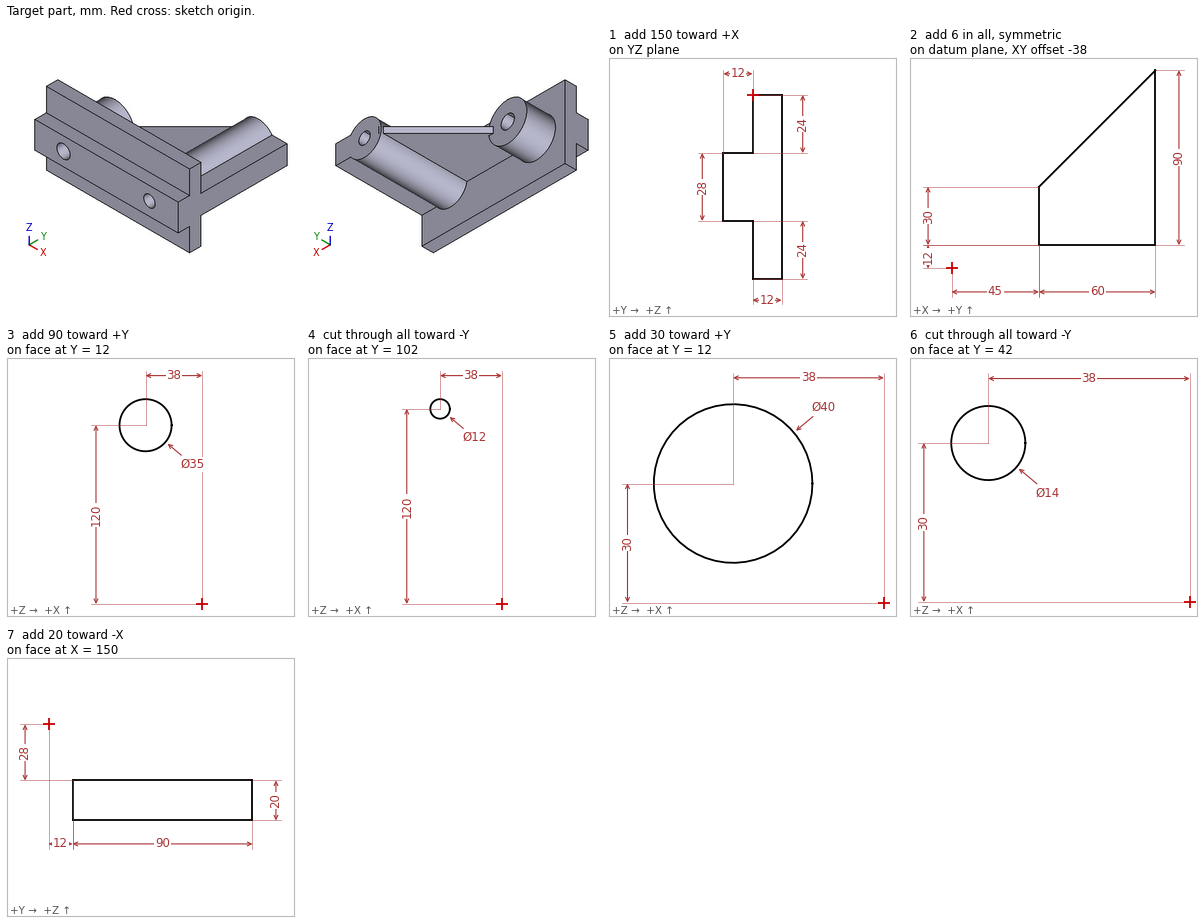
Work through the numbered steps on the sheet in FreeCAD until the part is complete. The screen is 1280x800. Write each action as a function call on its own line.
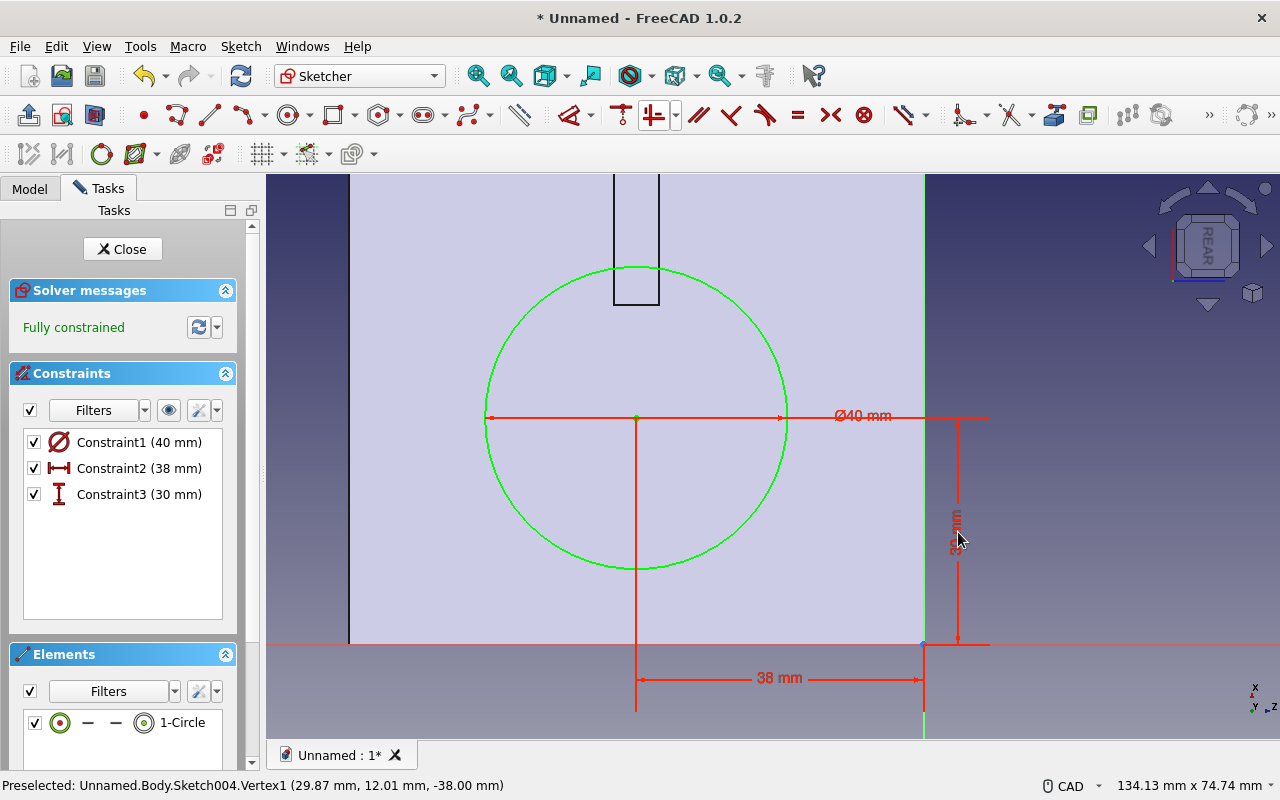
click(123, 249)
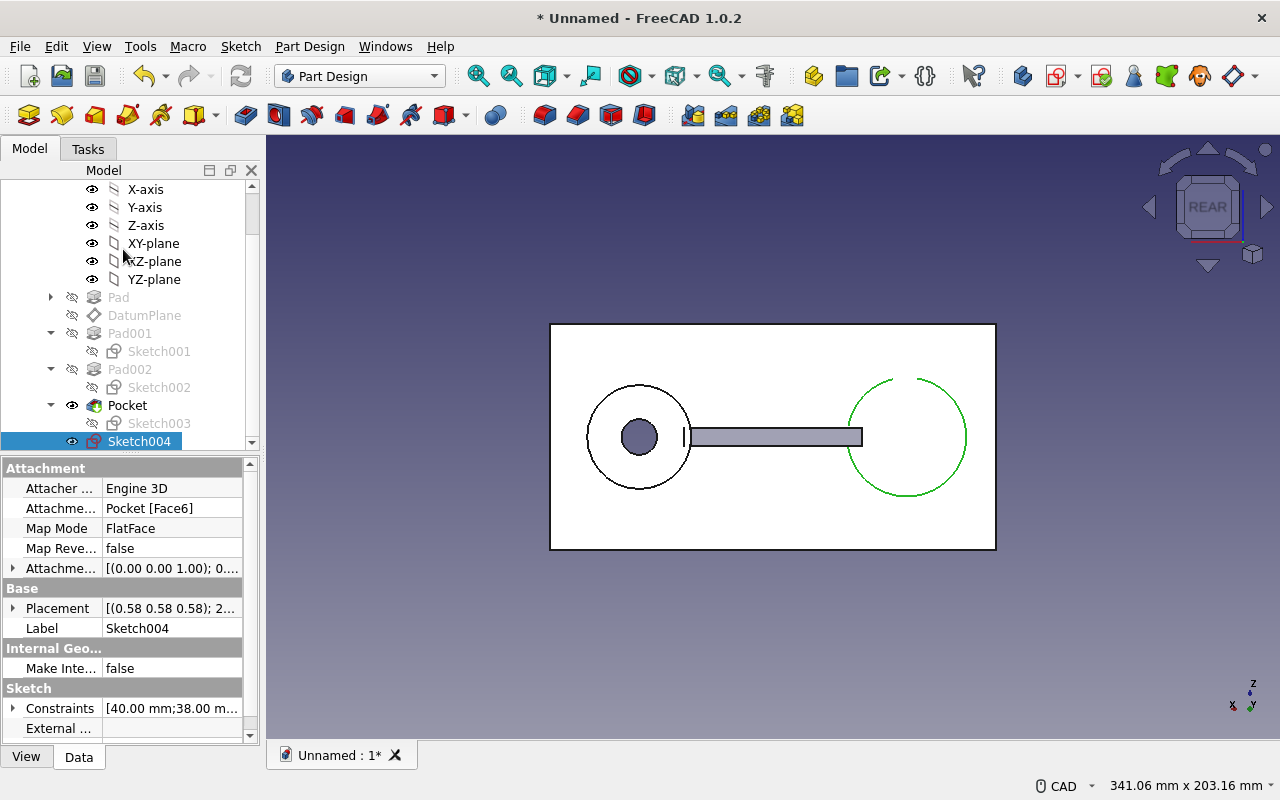
click(29, 116)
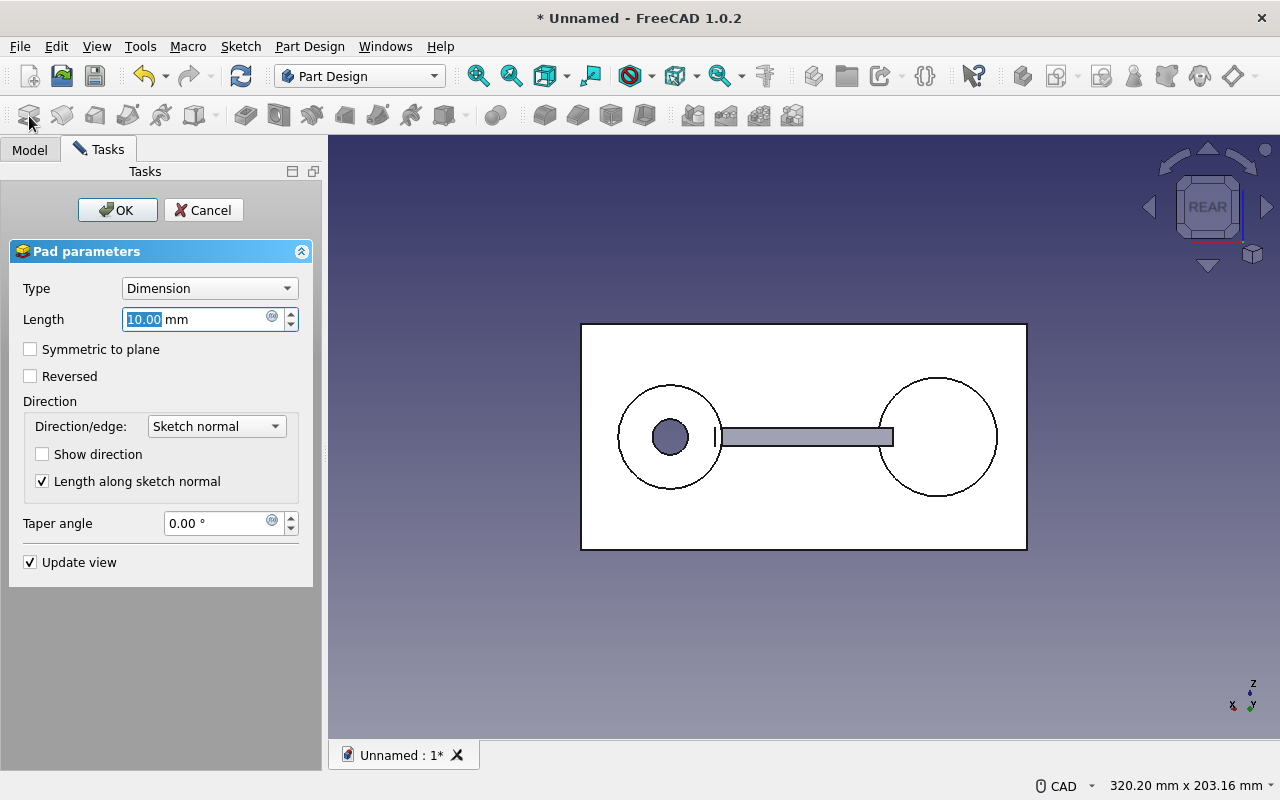
text(30)
key(Tab)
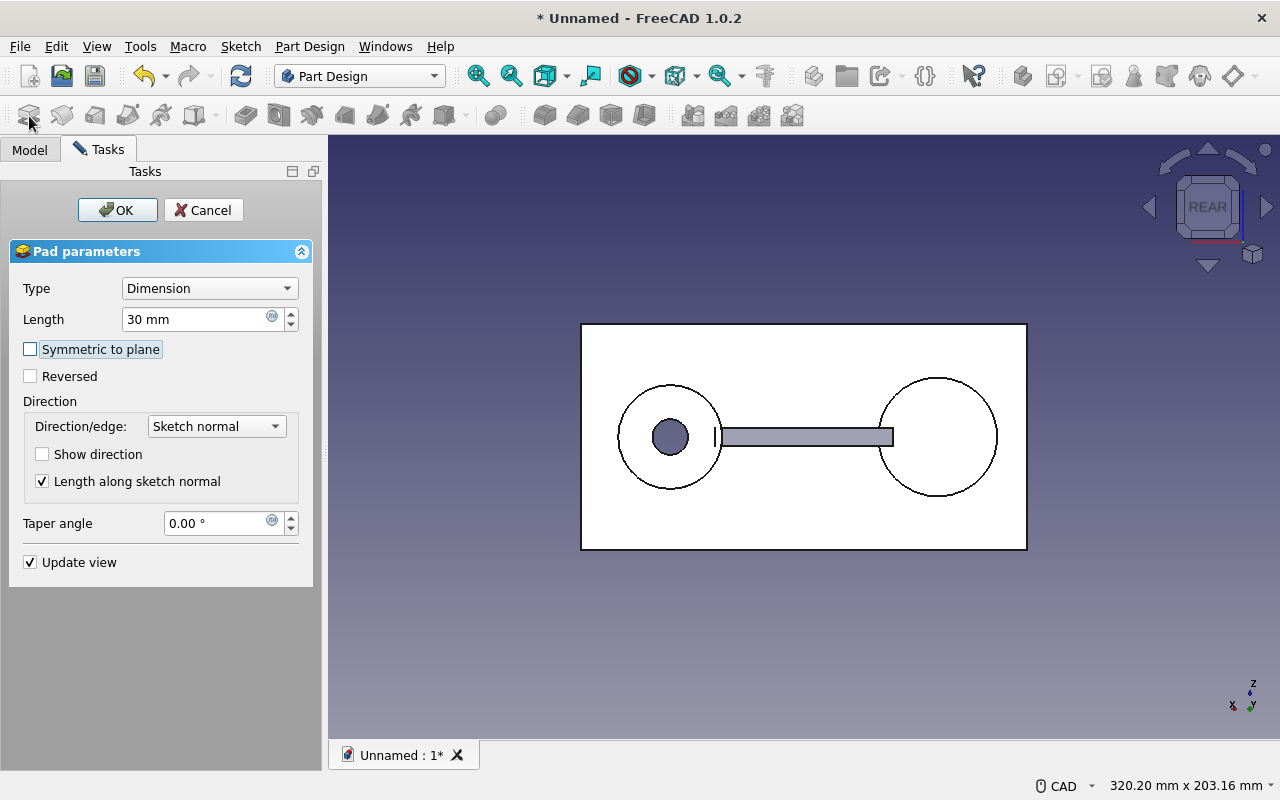
click(118, 210)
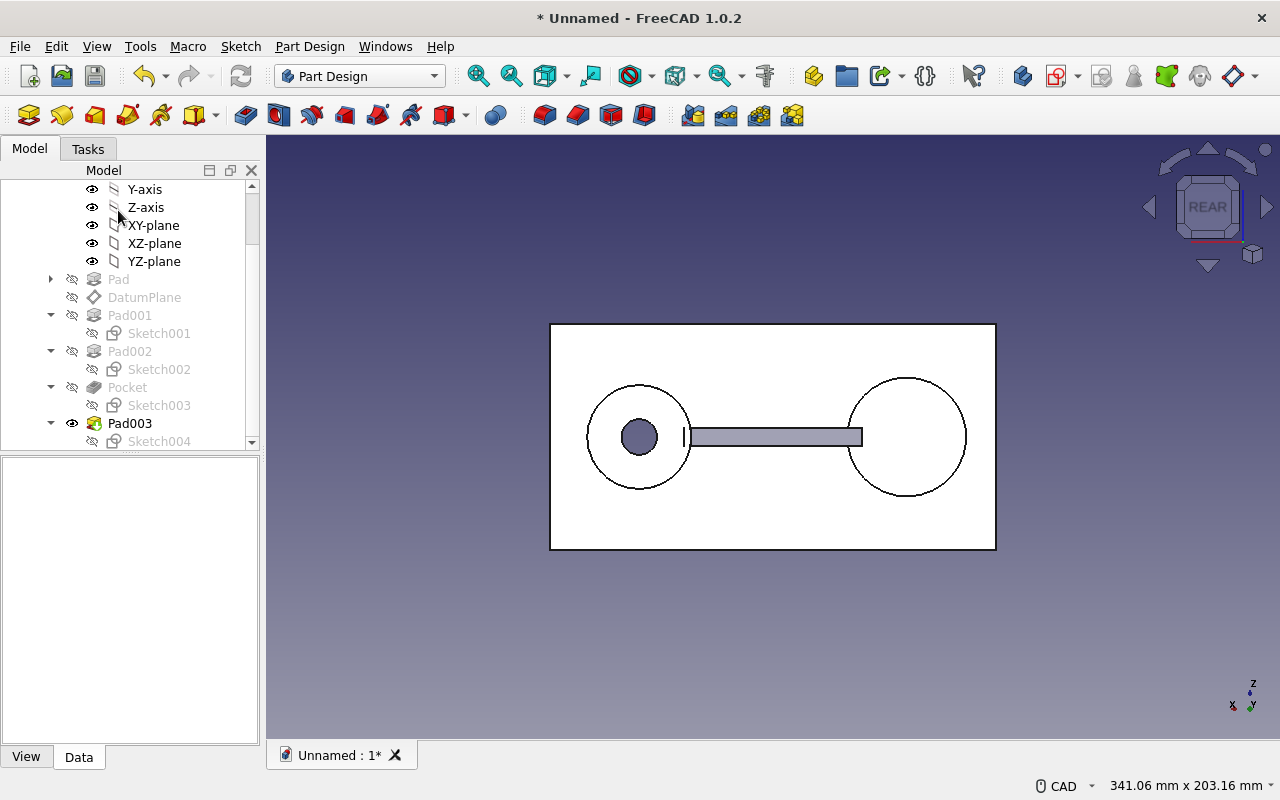
click(479, 76)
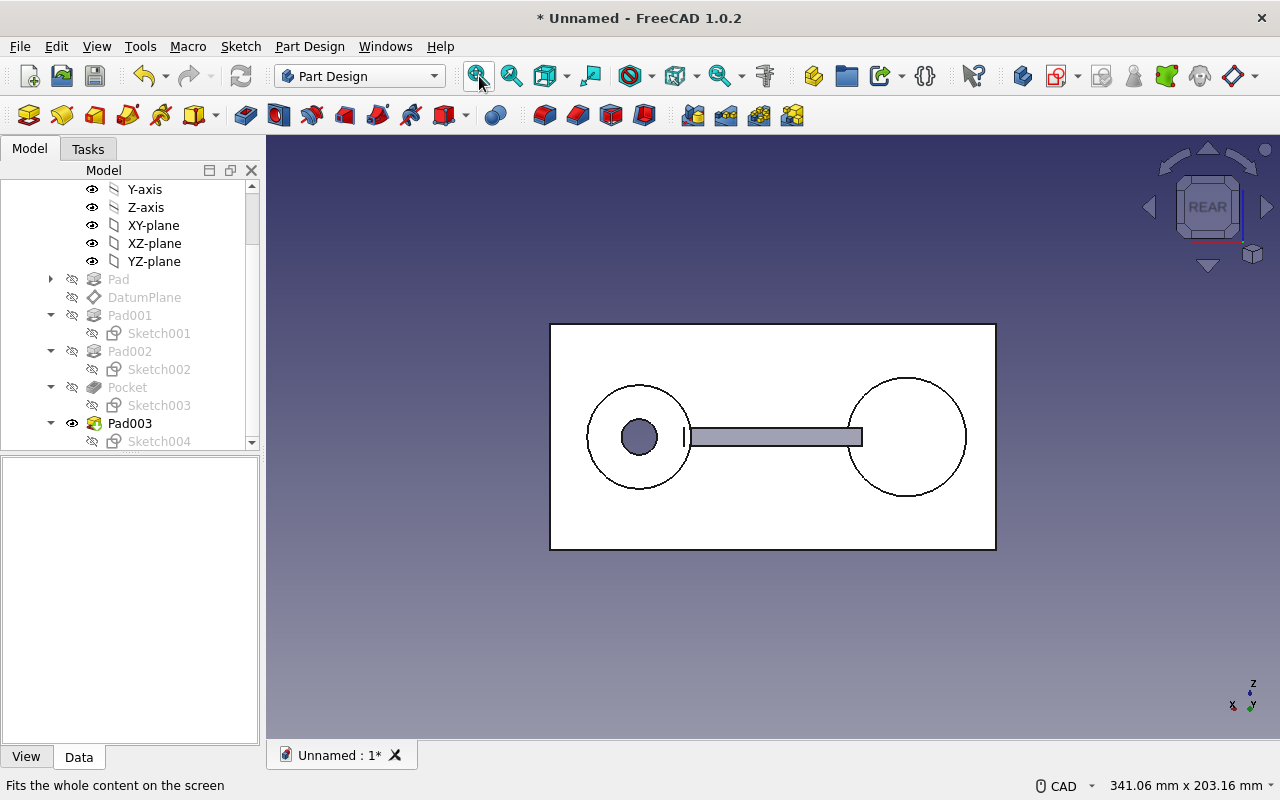
click(907, 436)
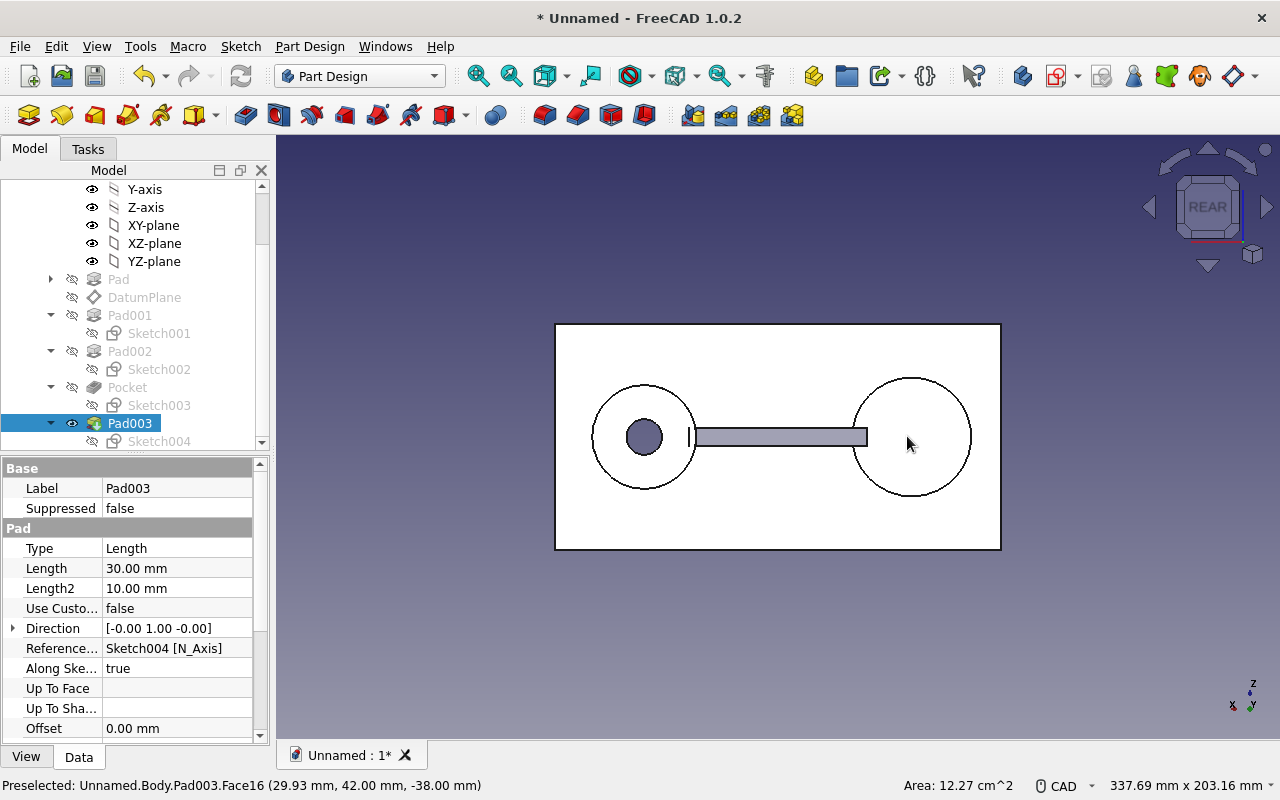
click(1056, 76)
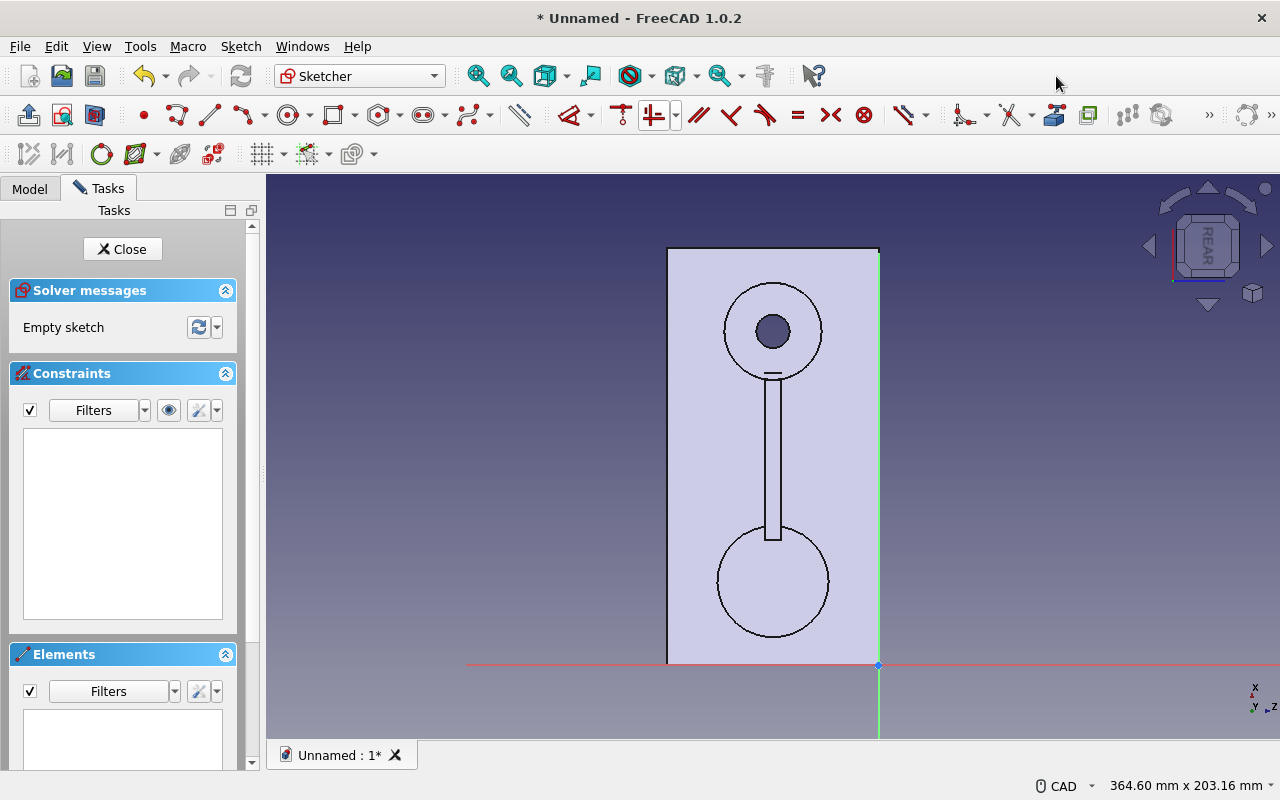
scroll(782, 597, up, 11)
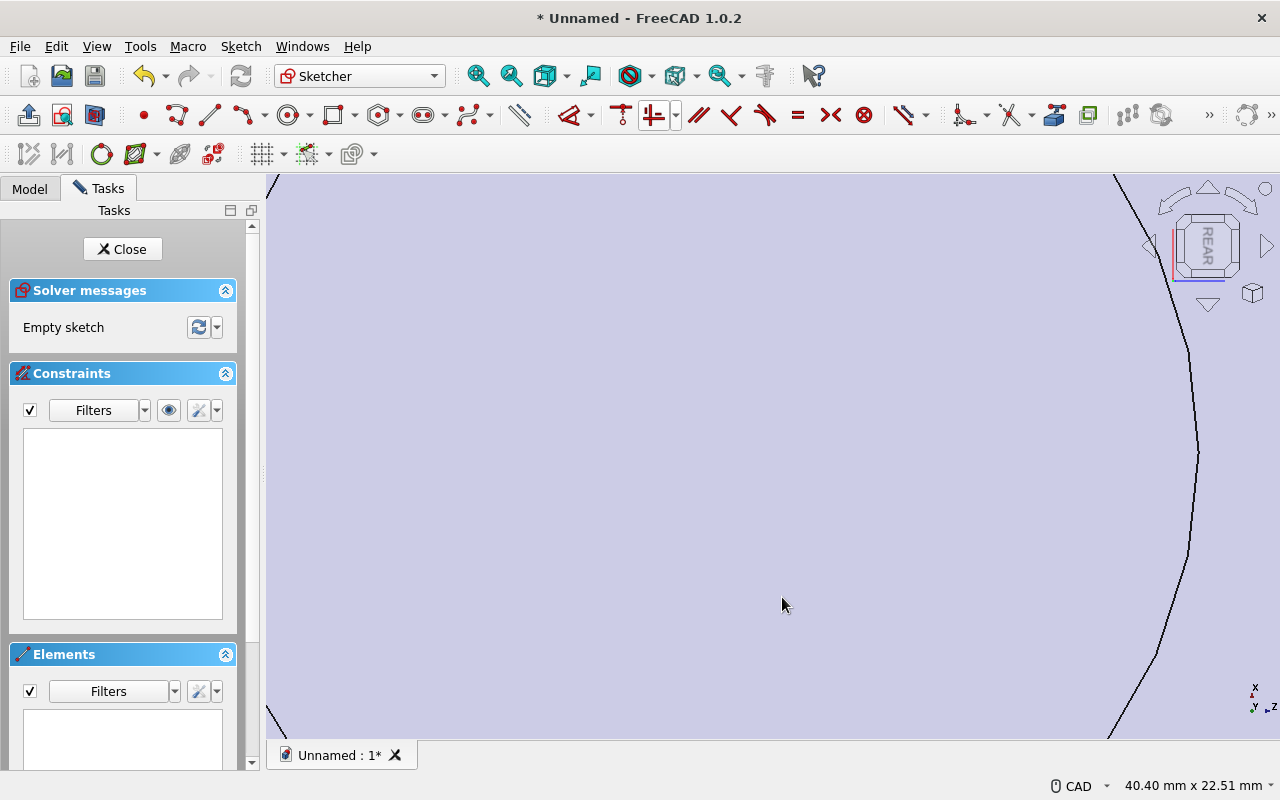
click(288, 116)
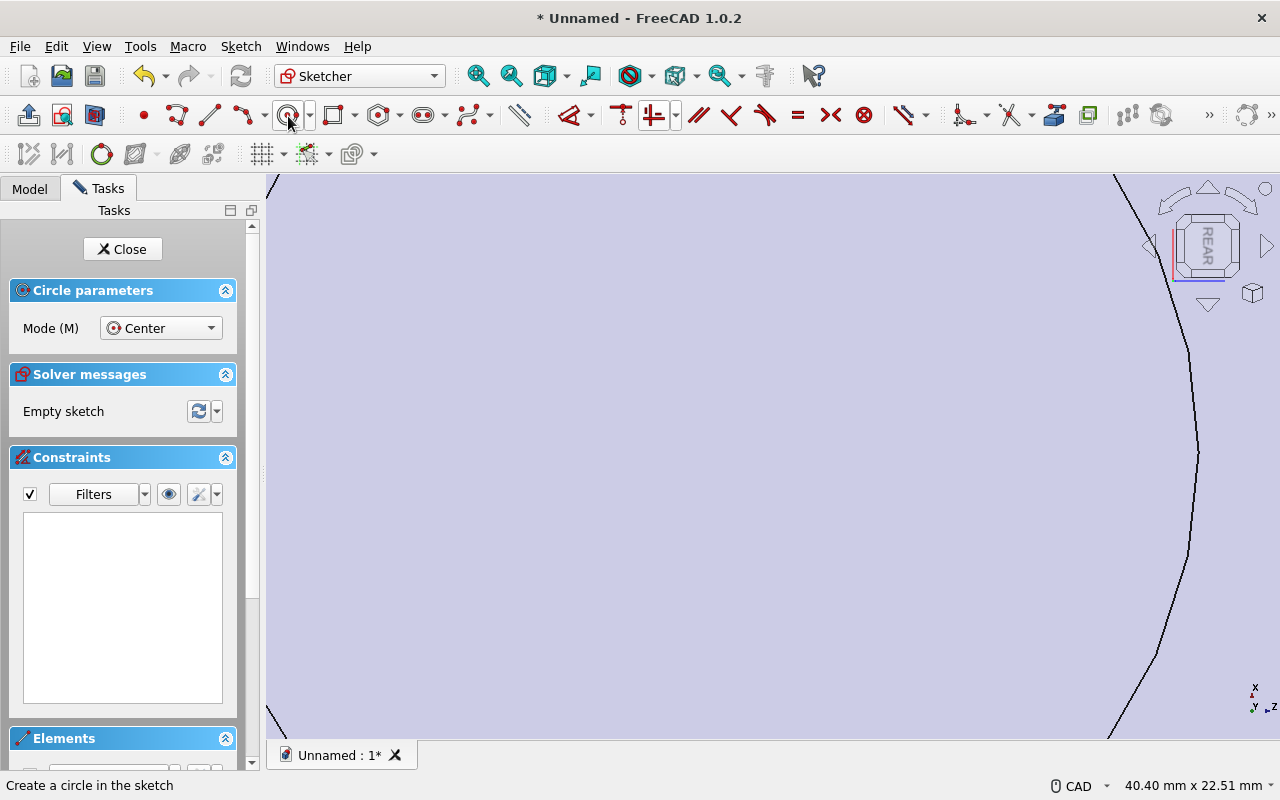
click(697, 452)
move(821, 328)